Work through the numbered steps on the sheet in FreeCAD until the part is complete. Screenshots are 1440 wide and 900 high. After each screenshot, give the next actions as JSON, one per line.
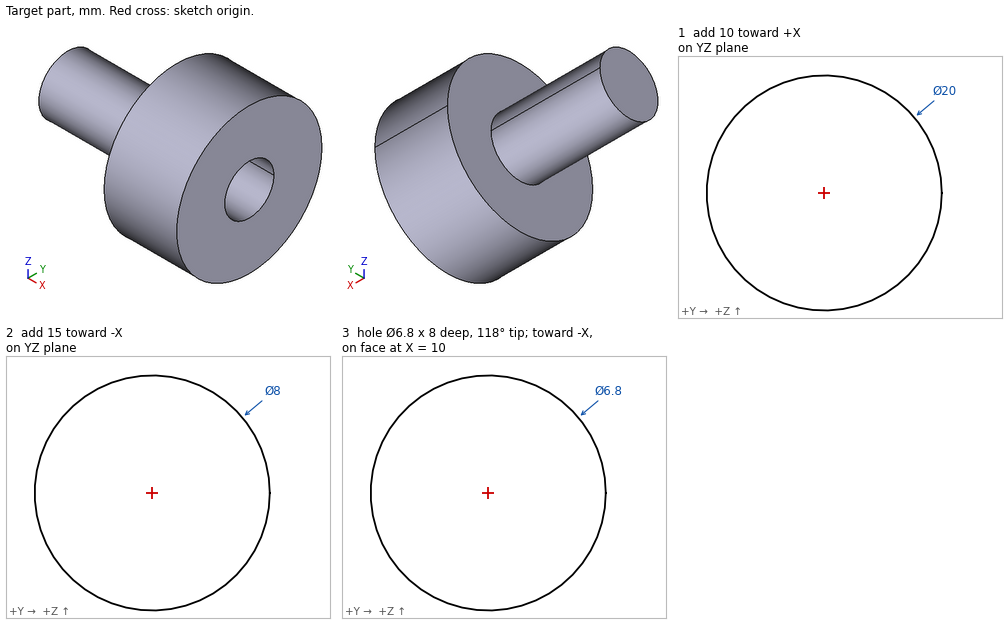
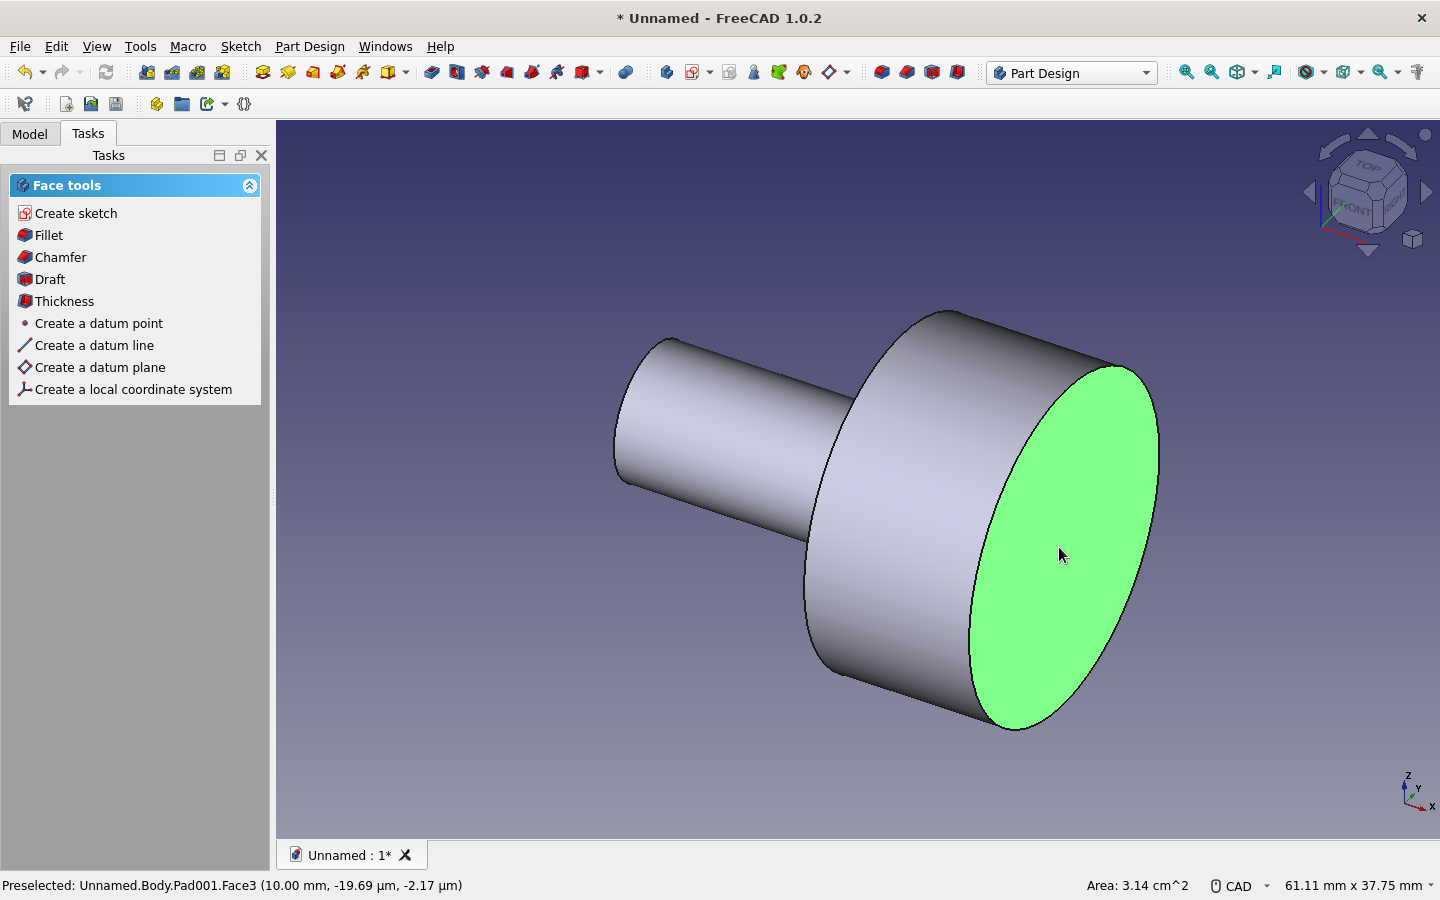
{"action": "left_click", "coordinate": [692, 72]}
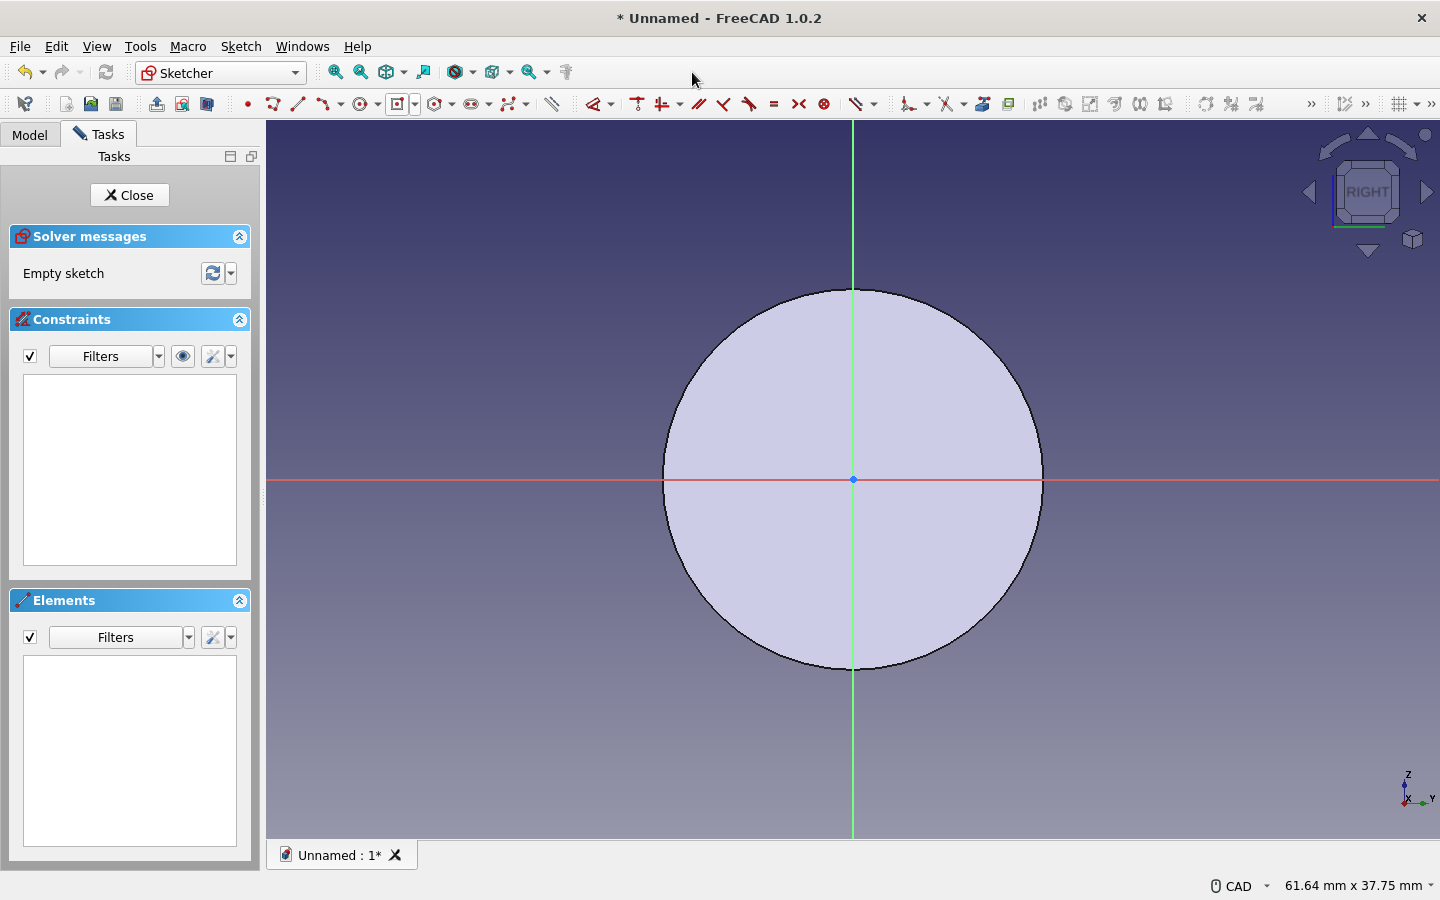
{"action": "scroll", "coordinate": [883, 479], "scroll_direction": "up", "scroll_amount": 6}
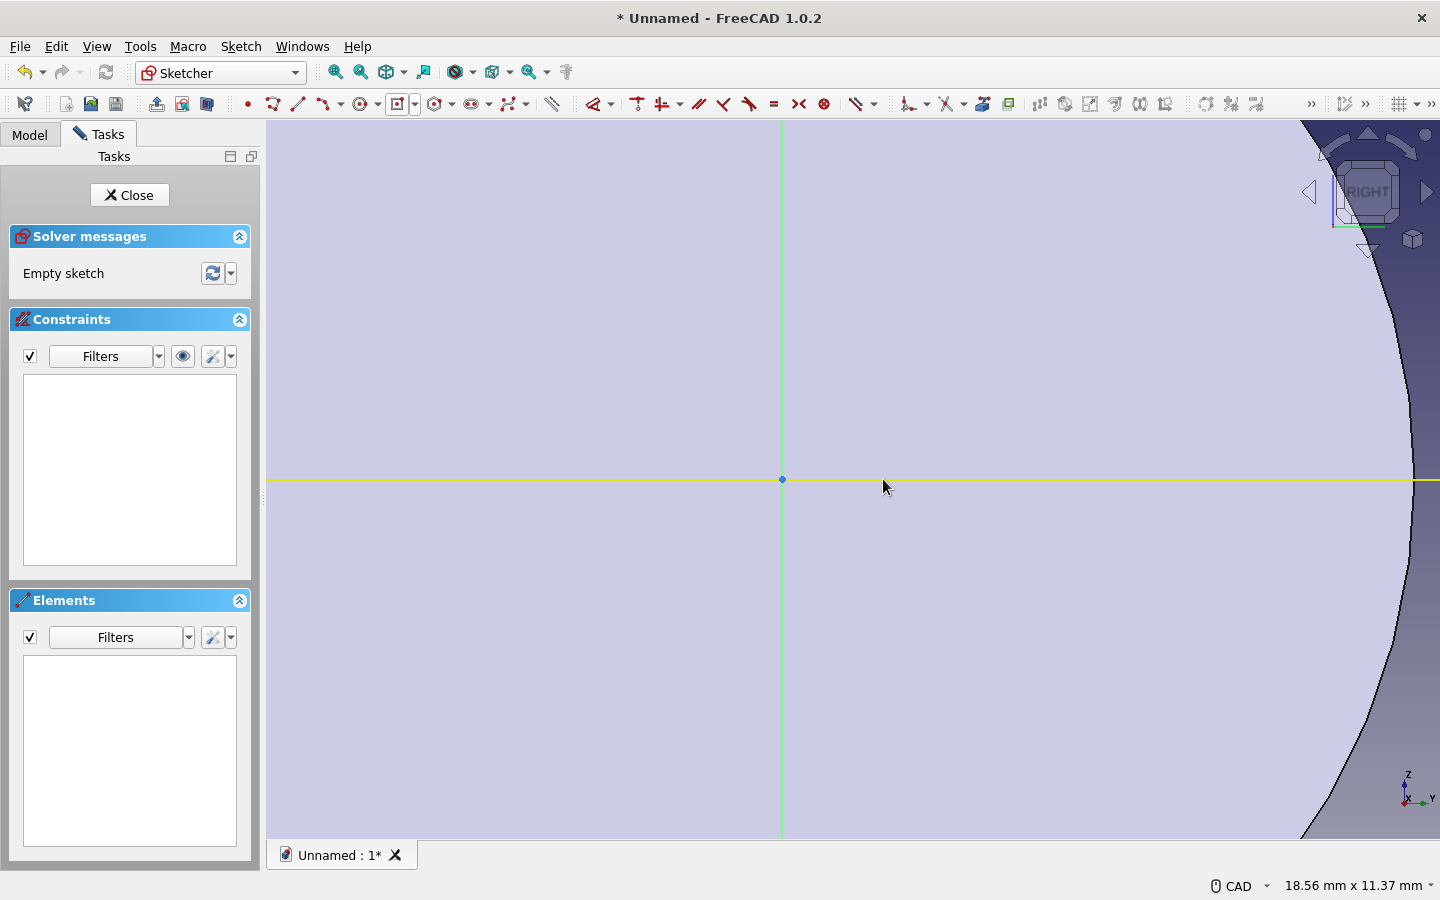
{"action": "left_click", "coordinate": [360, 104]}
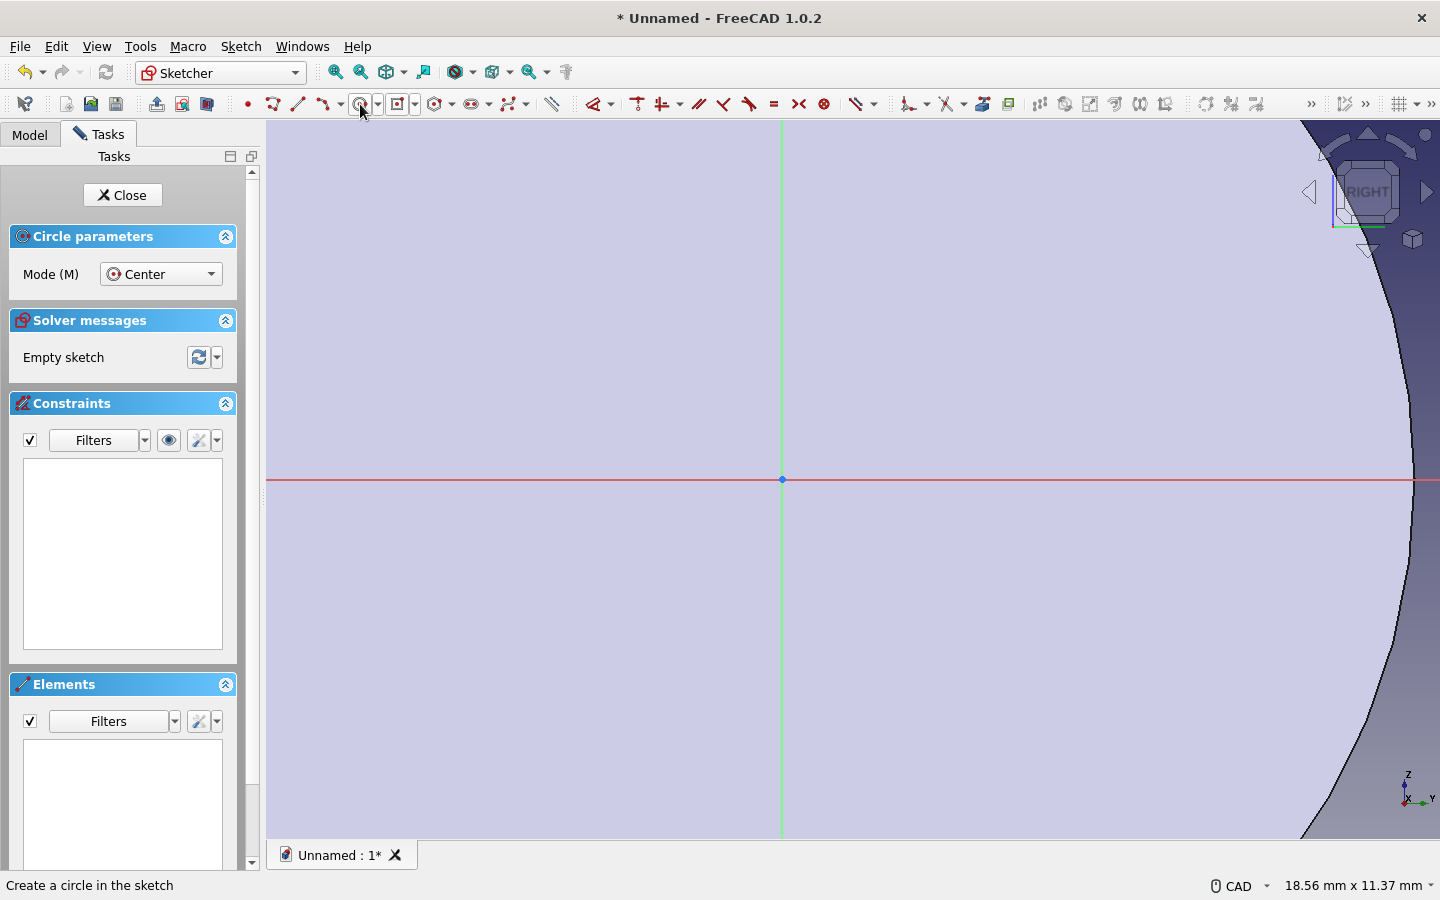
{"action": "left_click", "coordinate": [782, 479]}
{"action": "left_click", "coordinate": [934, 327]}
{"action": "key", "text": "Escape"}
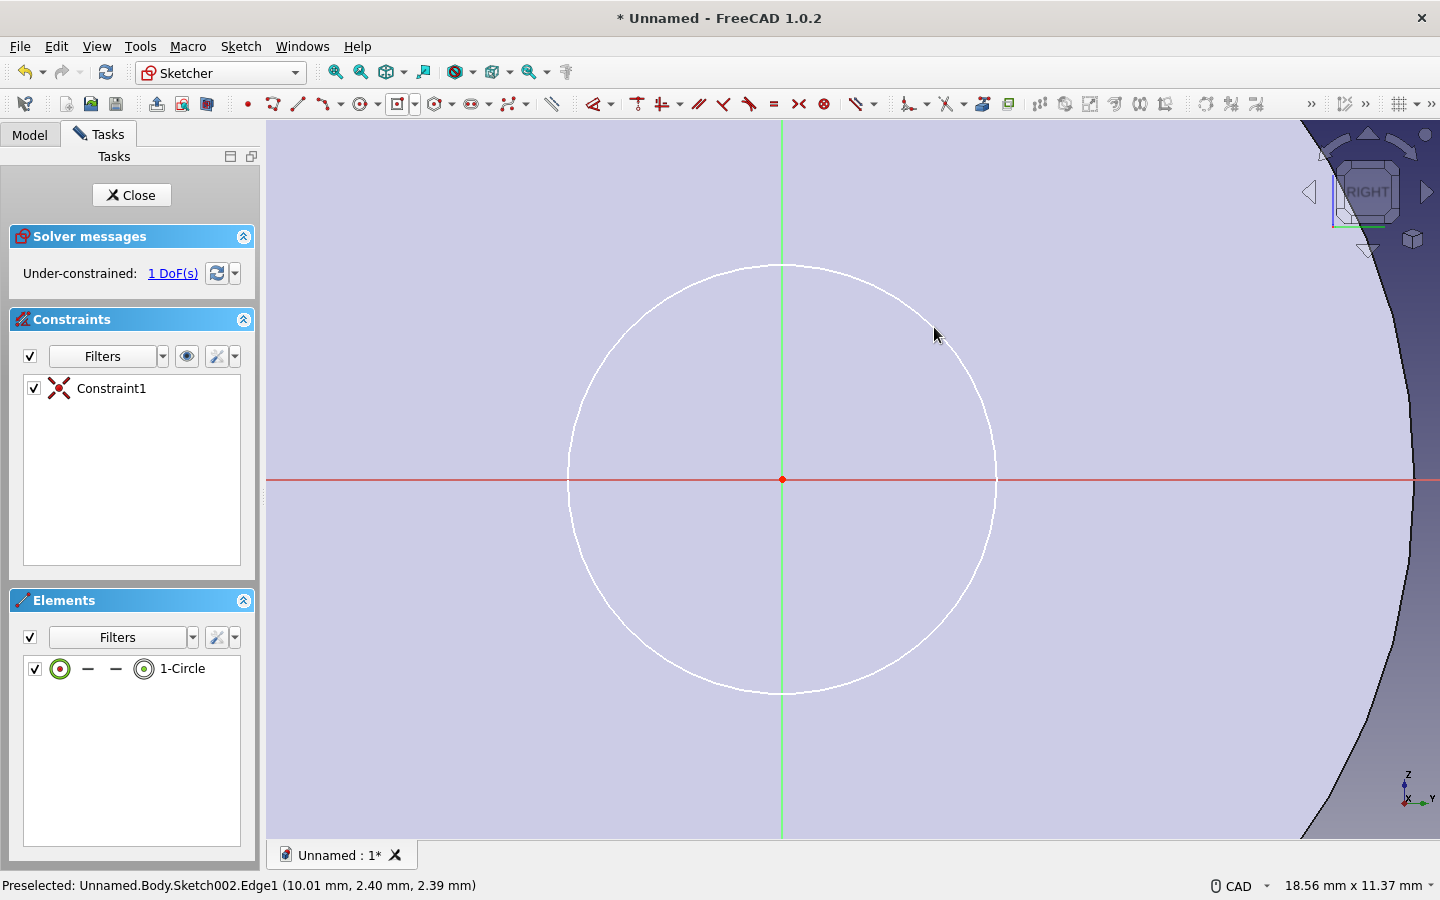
{"action": "left_click", "coordinate": [592, 104]}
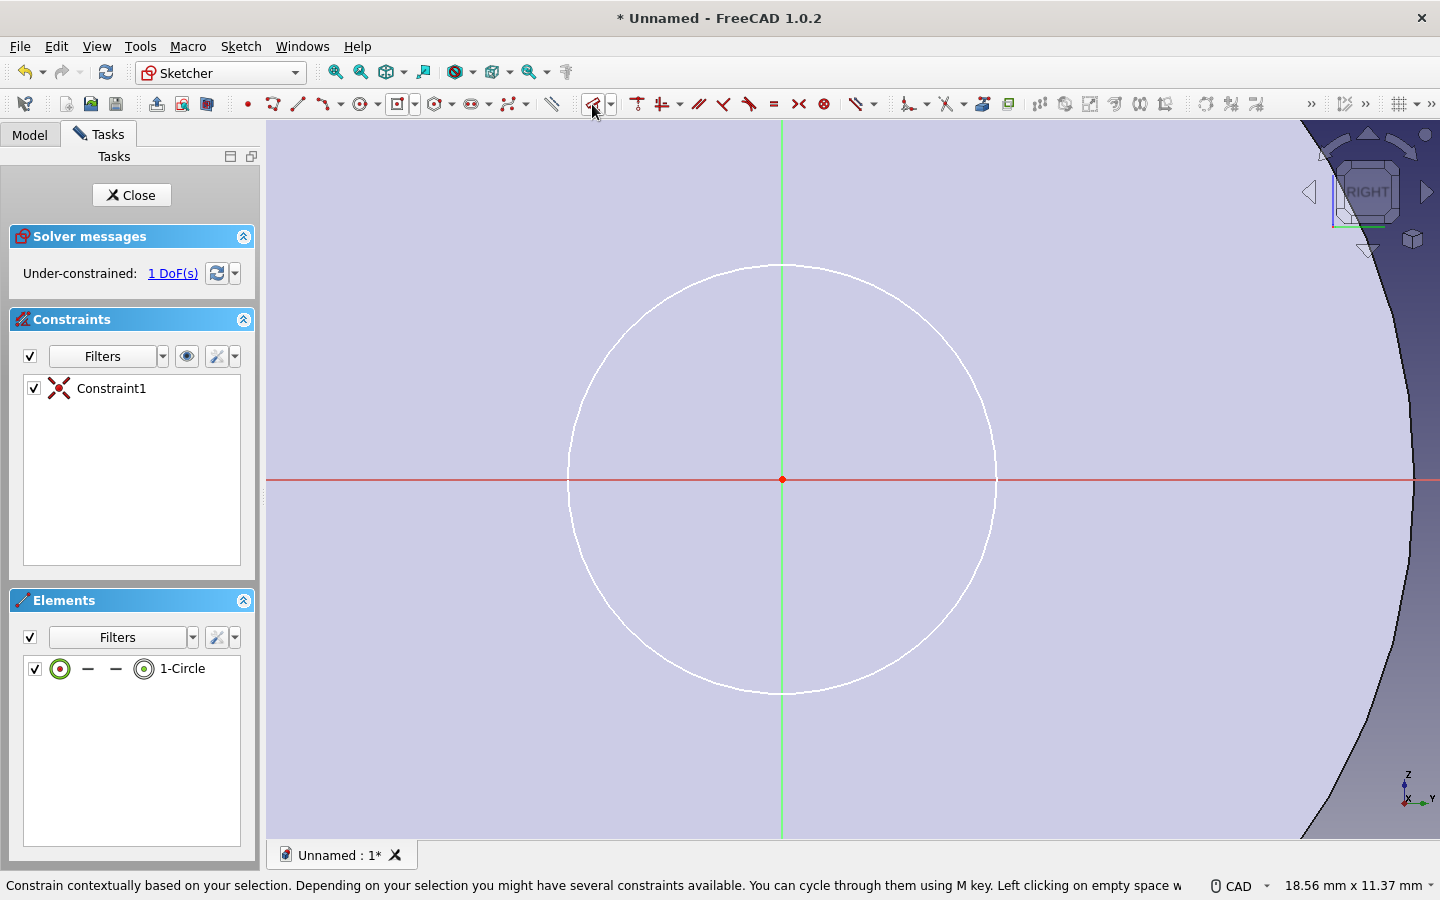
{"action": "left_click", "coordinate": [933, 327]}
{"action": "left_click", "coordinate": [956, 304]}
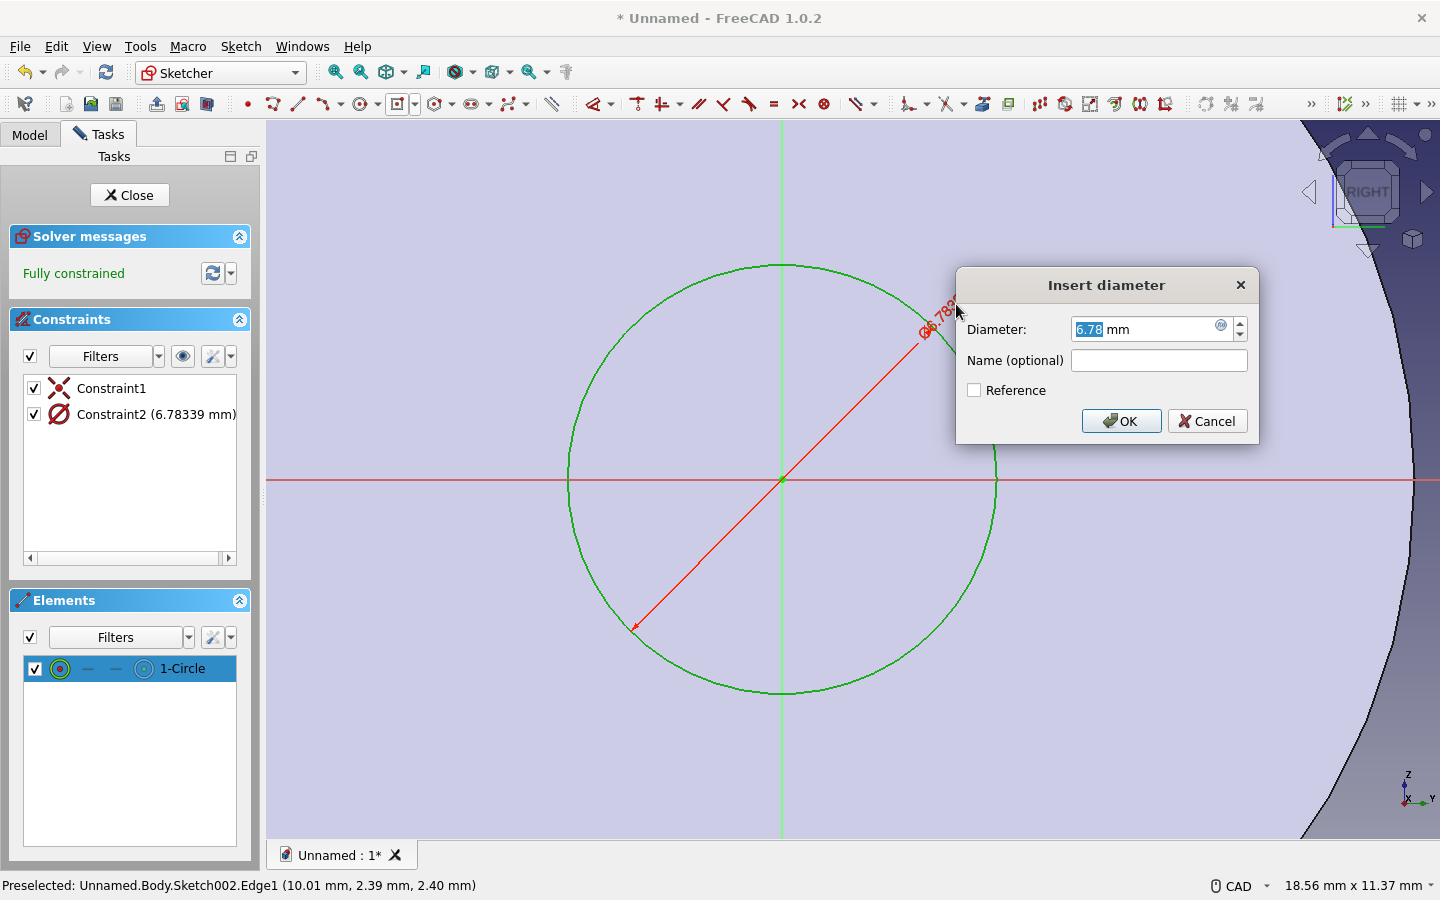
{"action": "type", "text": "6.8"}
{"action": "key", "text": "Return"}
{"action": "key", "text": "Escape"}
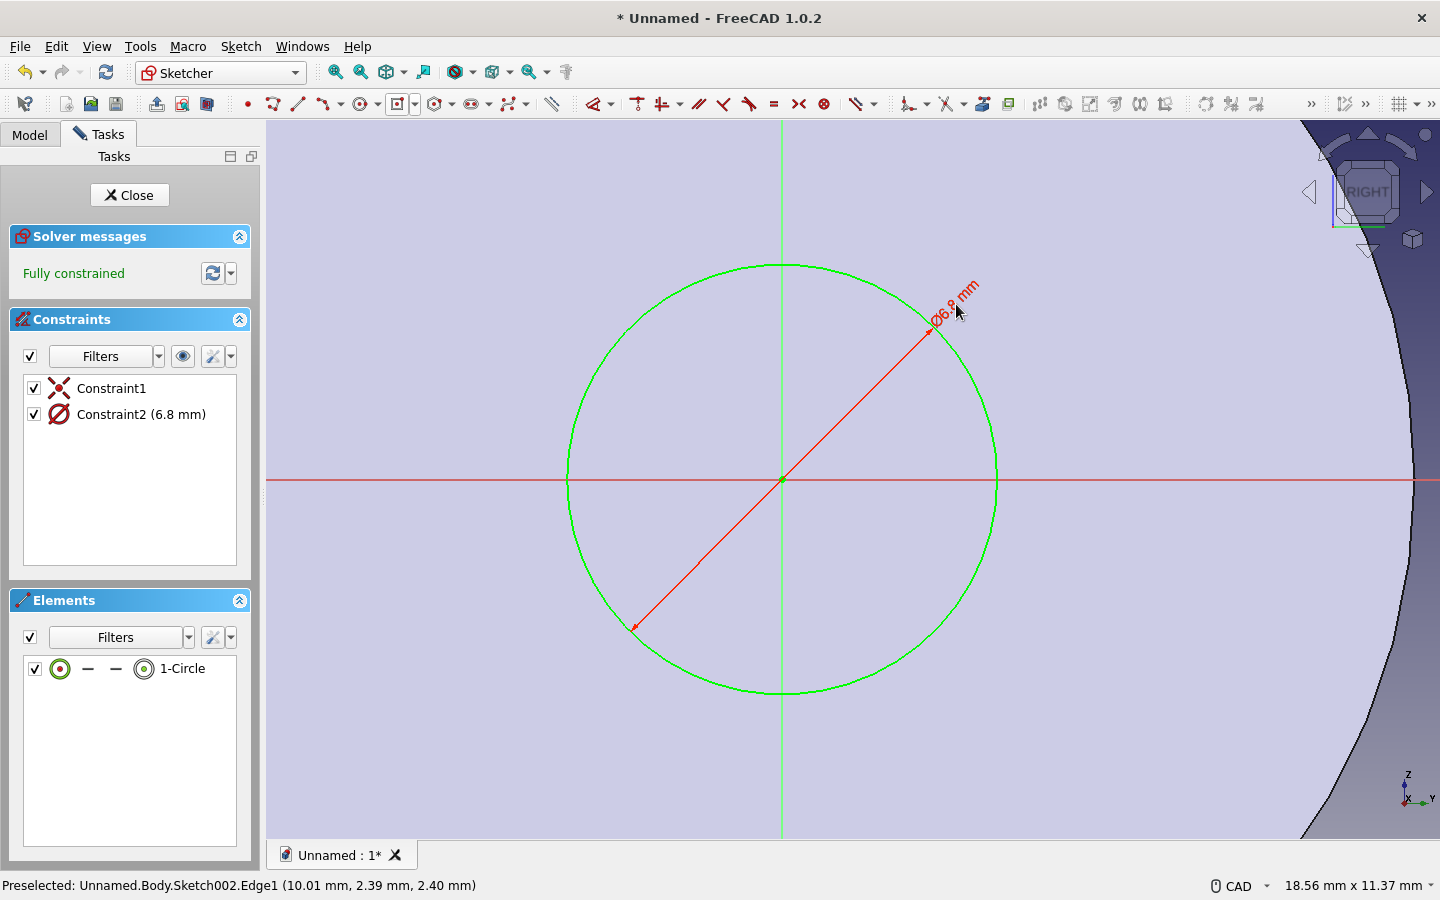
{"action": "left_click", "coordinate": [130, 195]}